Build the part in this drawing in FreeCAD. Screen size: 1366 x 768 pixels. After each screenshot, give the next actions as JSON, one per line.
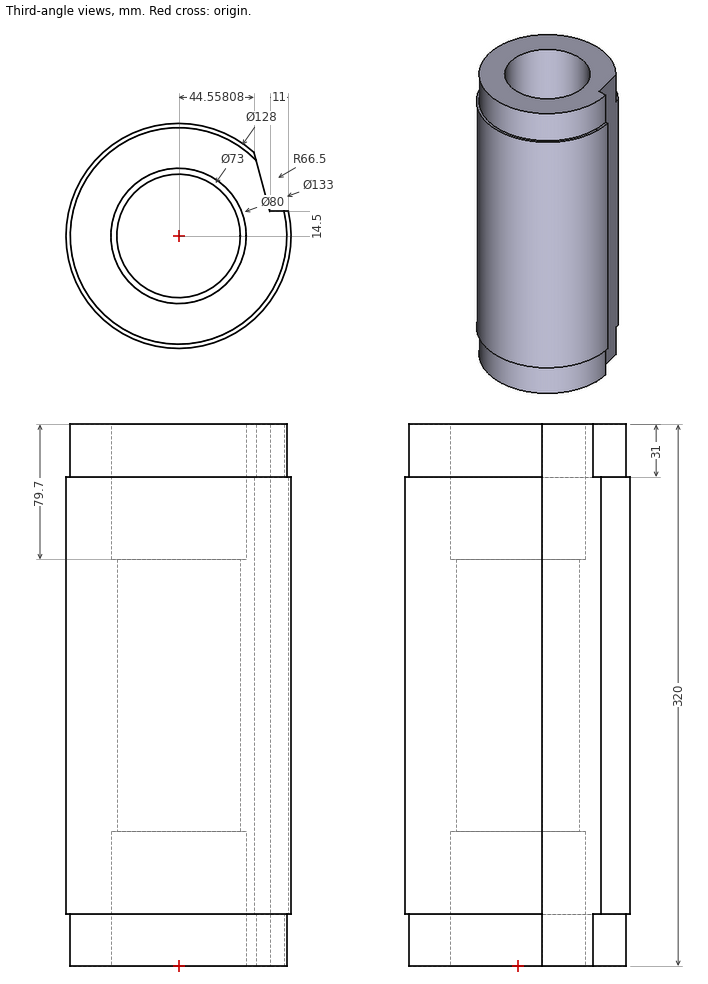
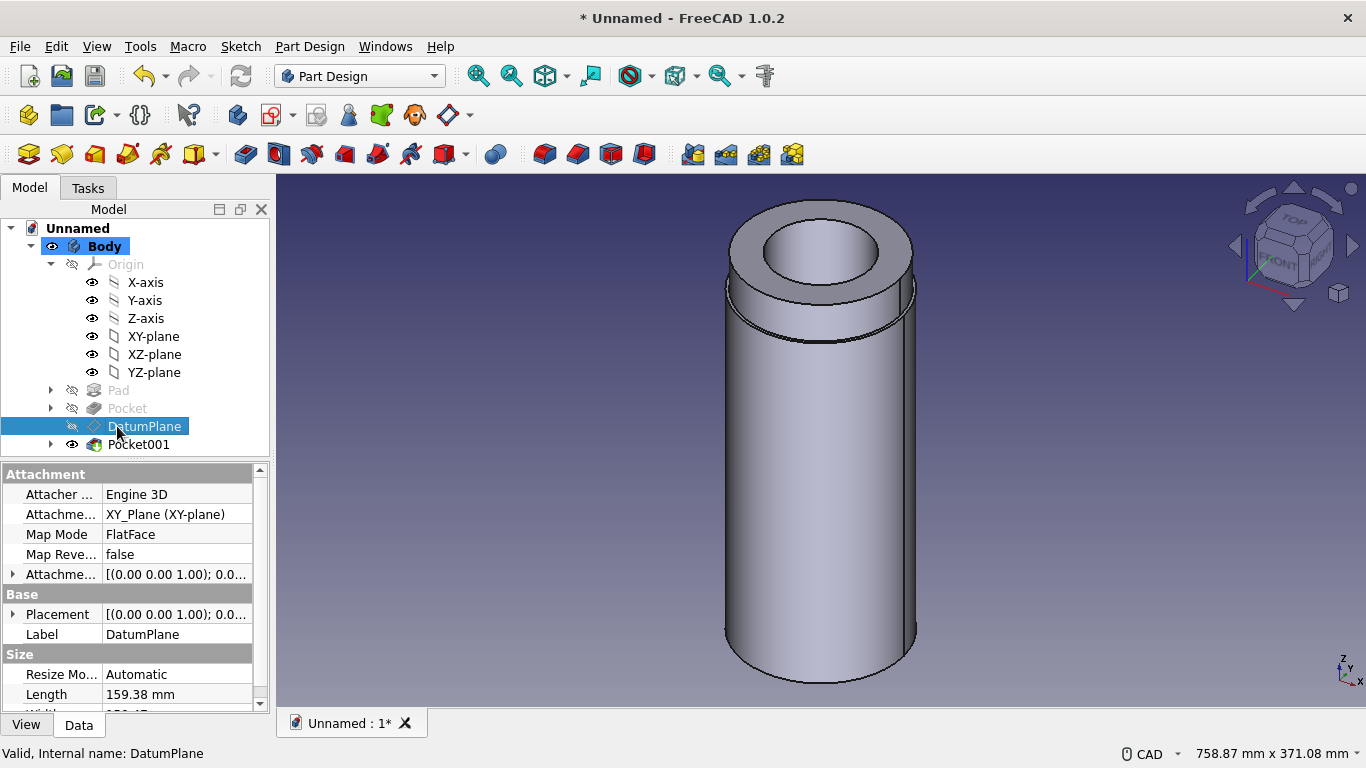
{"action": "left_click", "coordinate": [137, 336]}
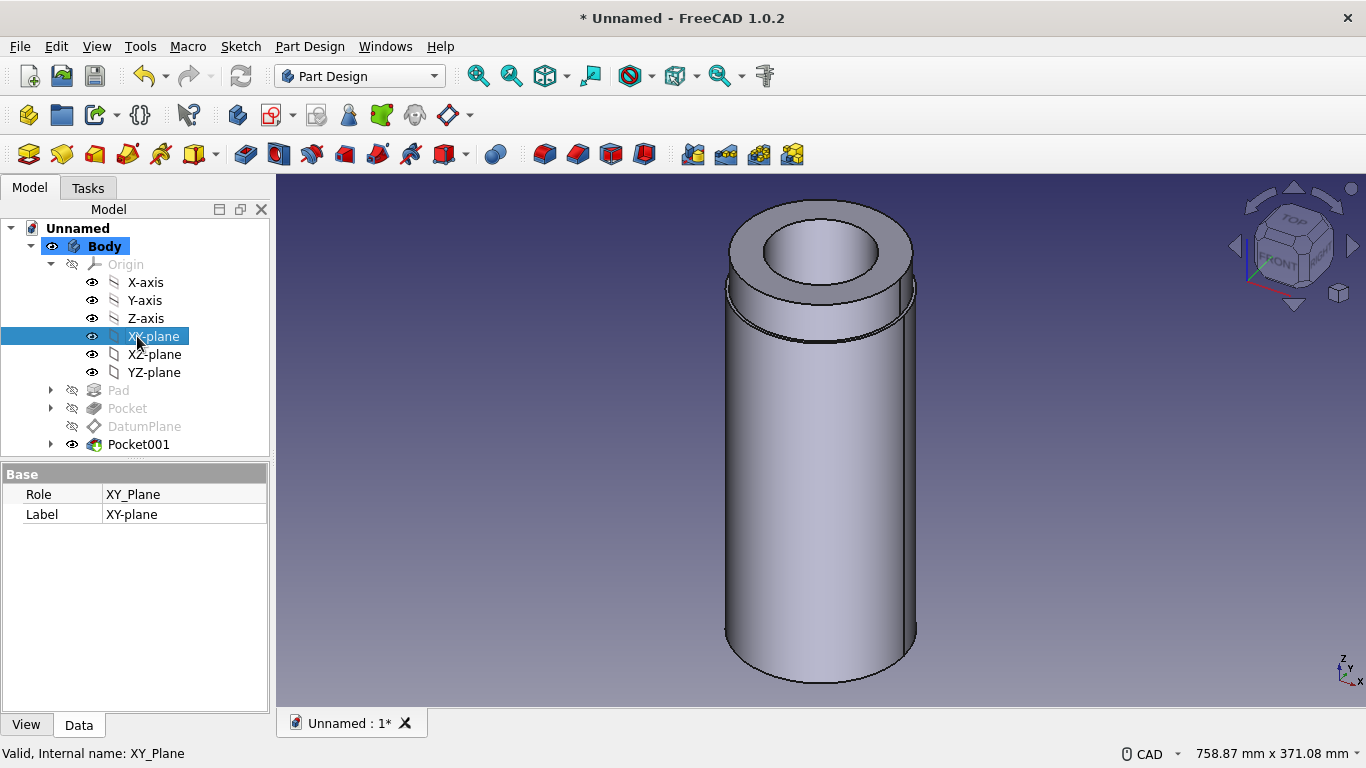
{"action": "left_click", "coordinate": [448, 116]}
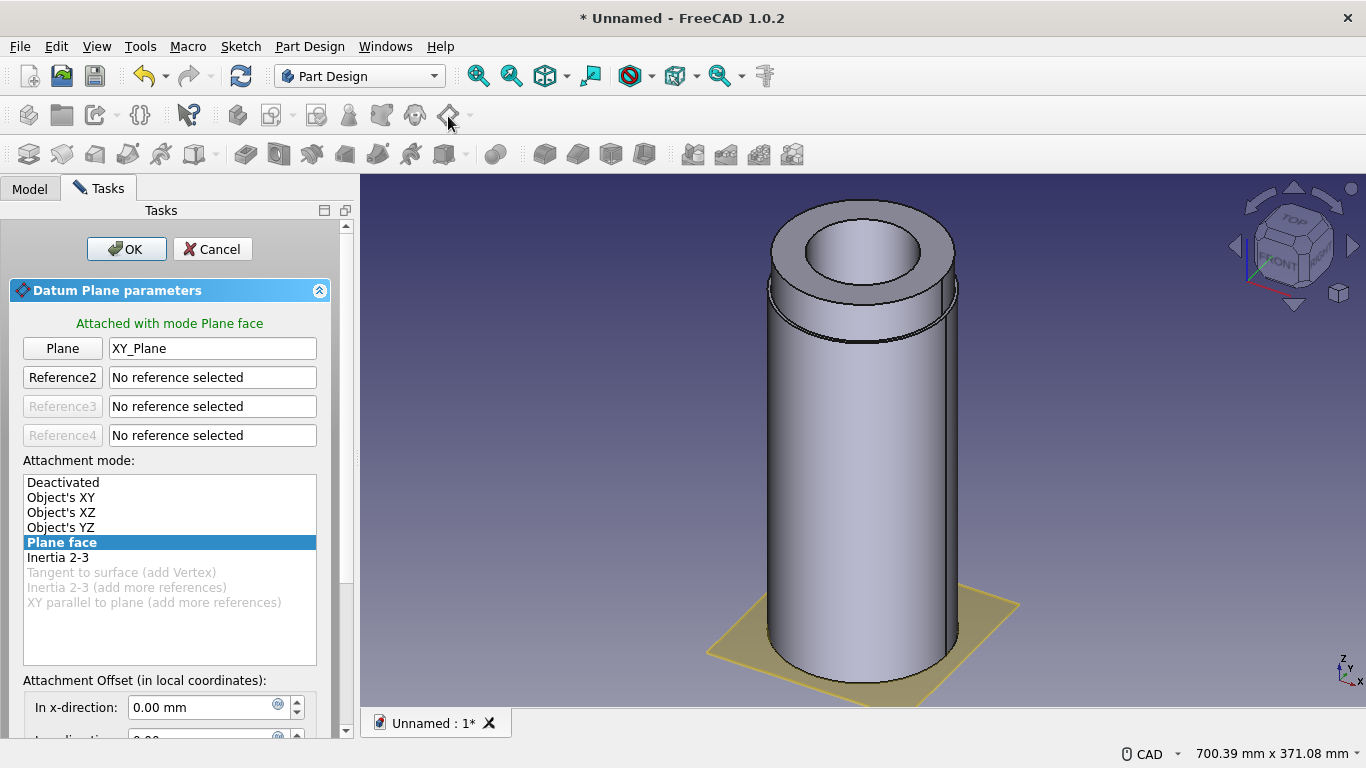
{"action": "scroll", "coordinate": [346, 479], "scroll_direction": "down", "scroll_amount": 2}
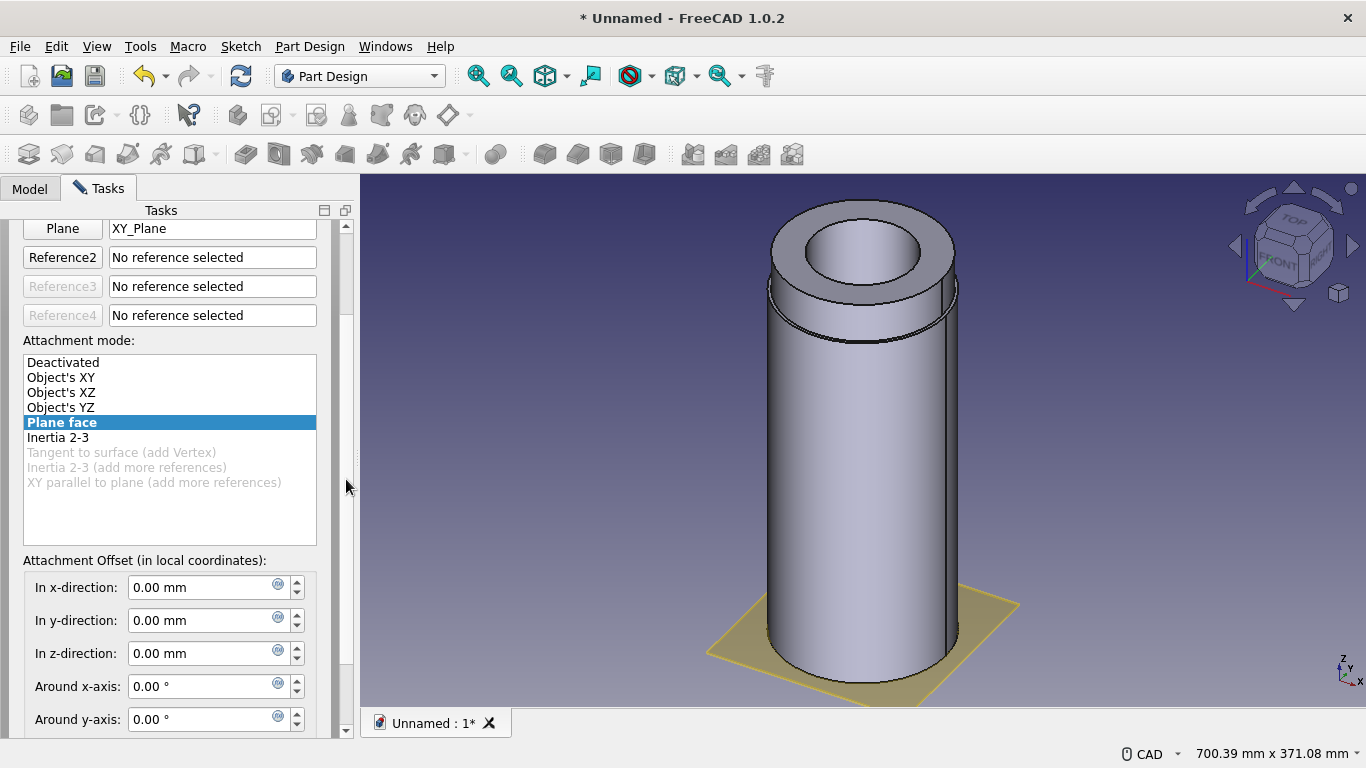
{"action": "triple_click", "coordinate": [210, 654]}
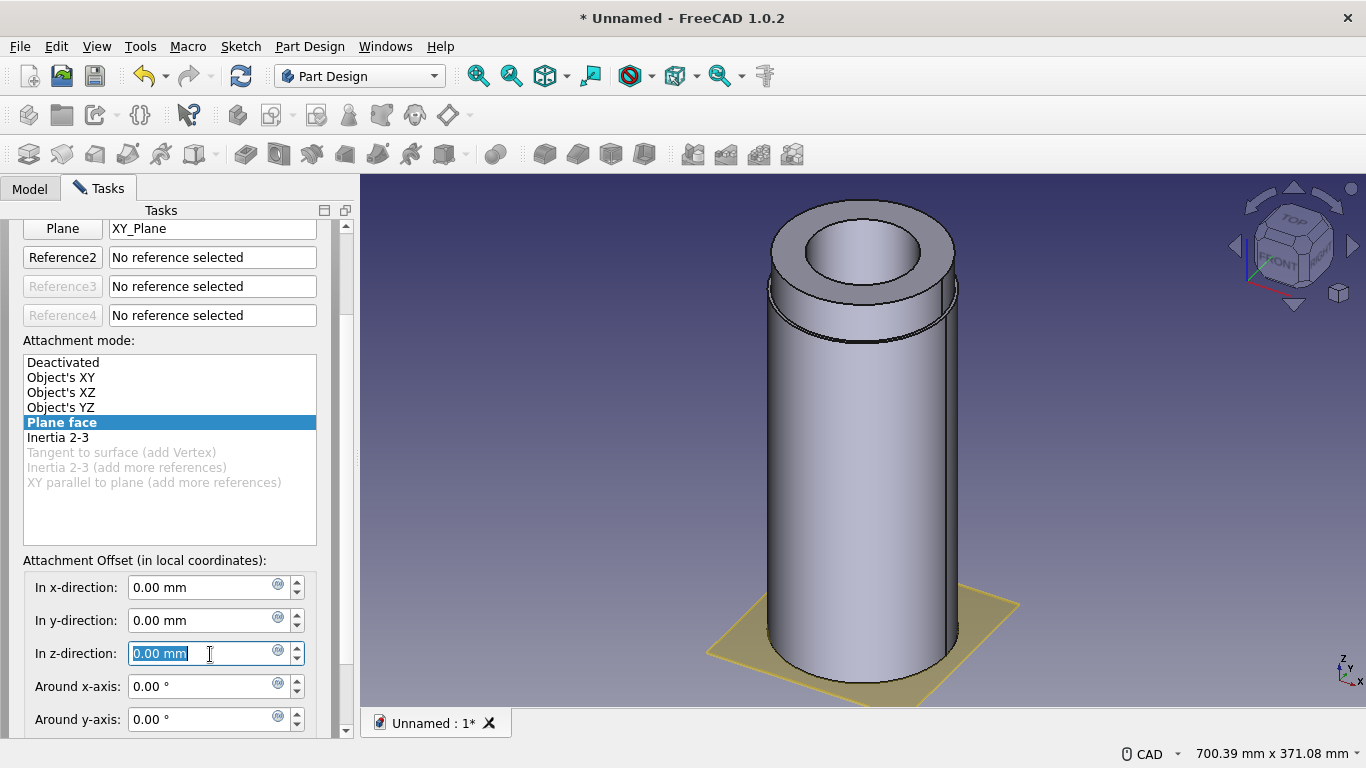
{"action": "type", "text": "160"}
{"action": "key", "text": "Tab"}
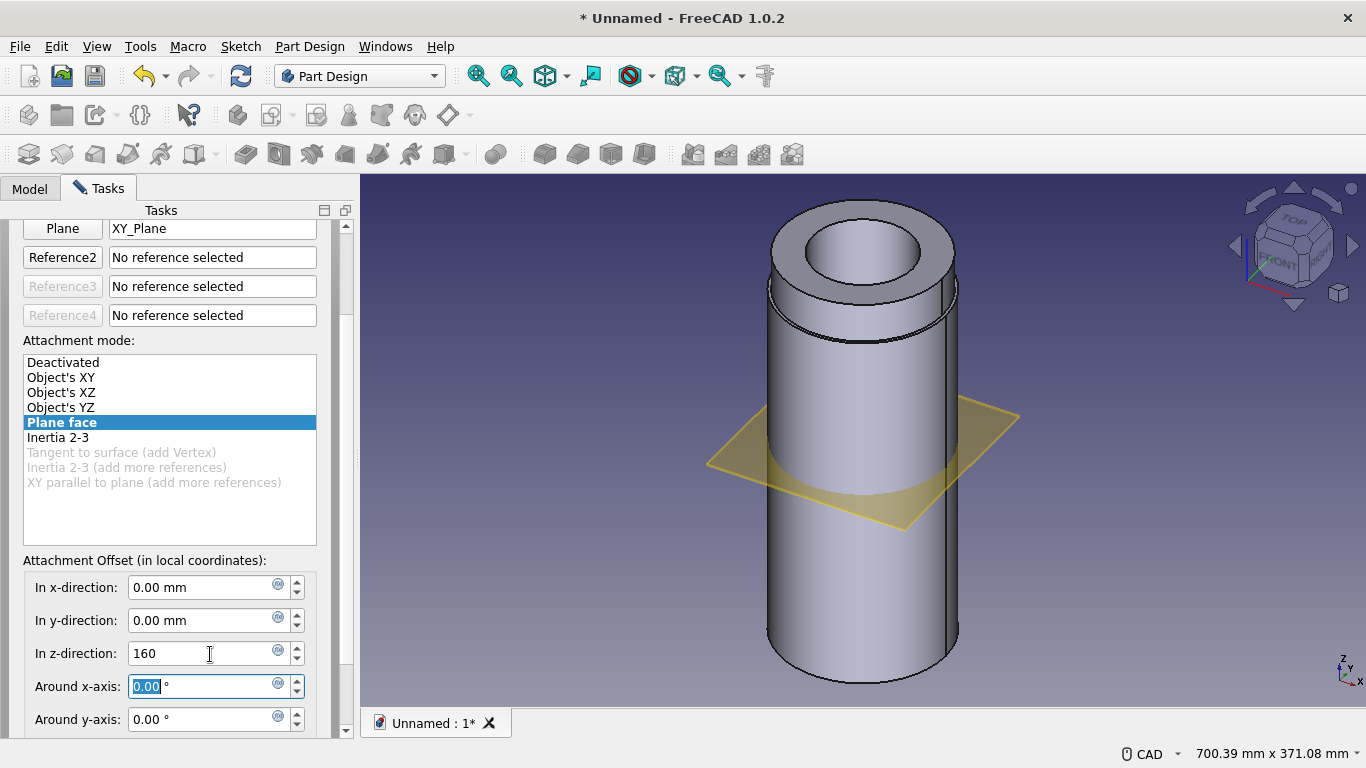
{"action": "scroll", "coordinate": [346, 479], "scroll_direction": "up", "scroll_amount": 3}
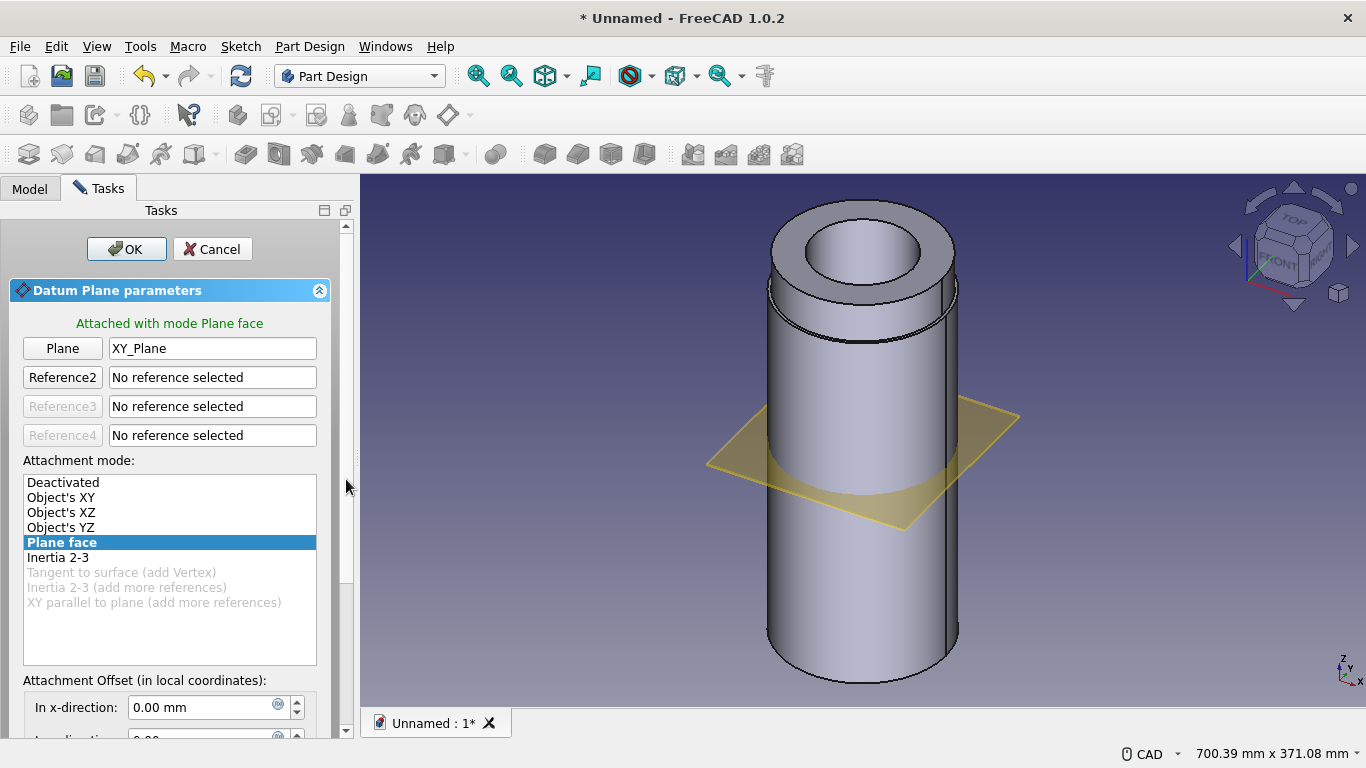
{"action": "left_click", "coordinate": [127, 249]}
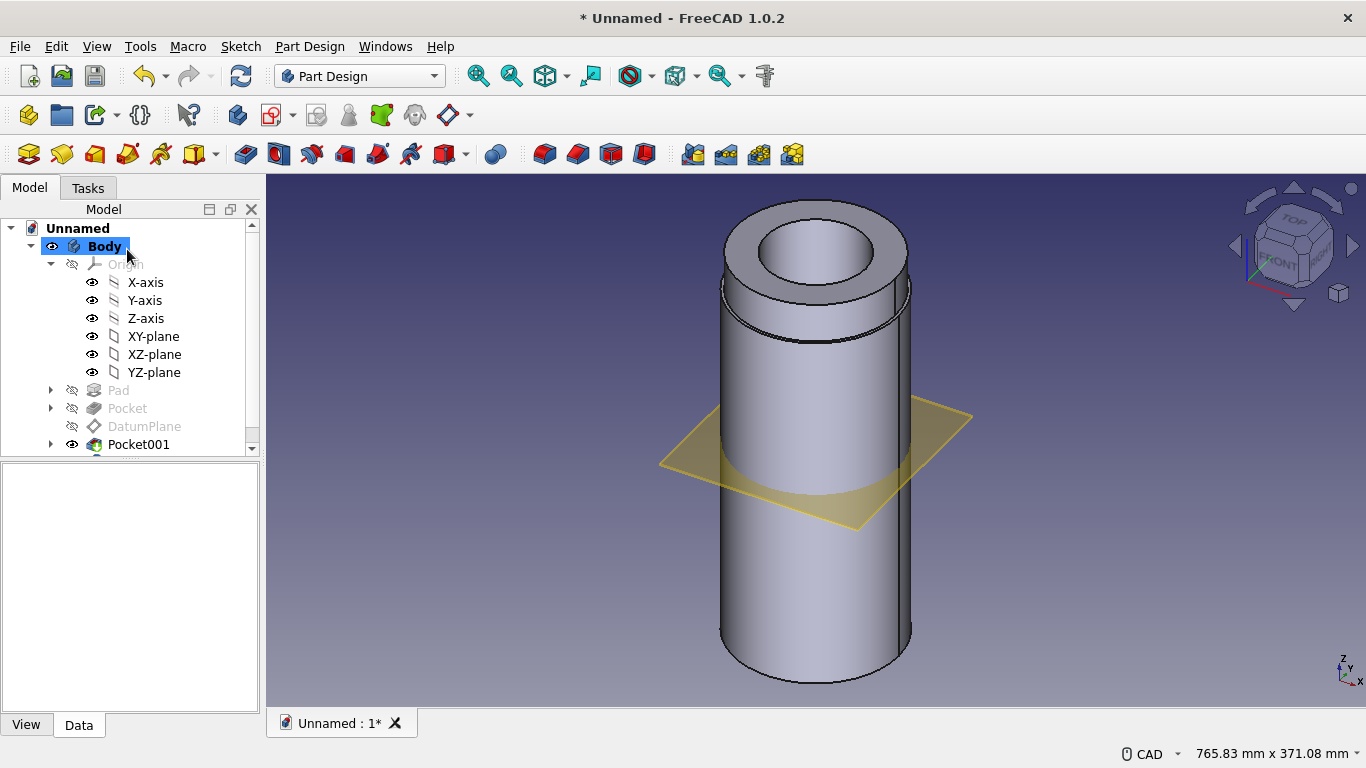
{"action": "left_click", "coordinate": [117, 408]}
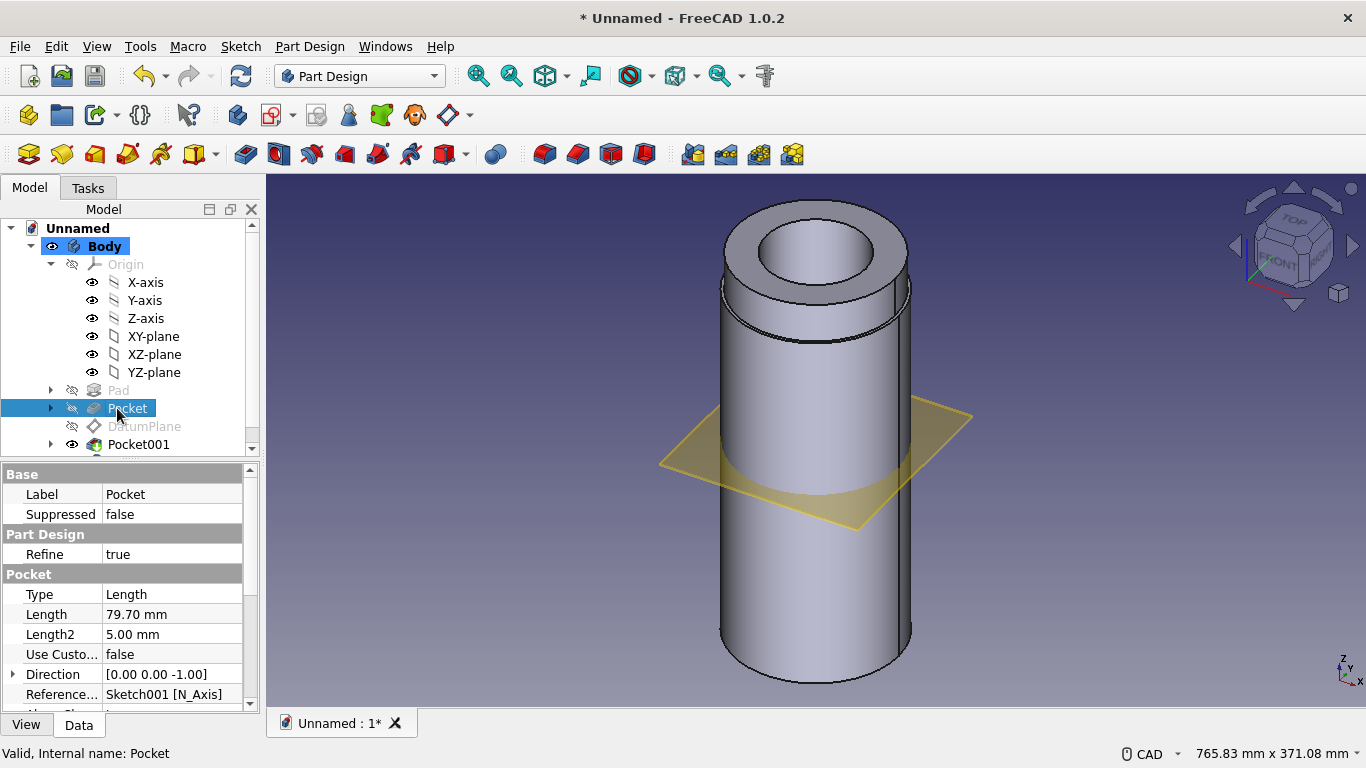
{"action": "left_click", "coordinate": [117, 444], "text": "ctrl"}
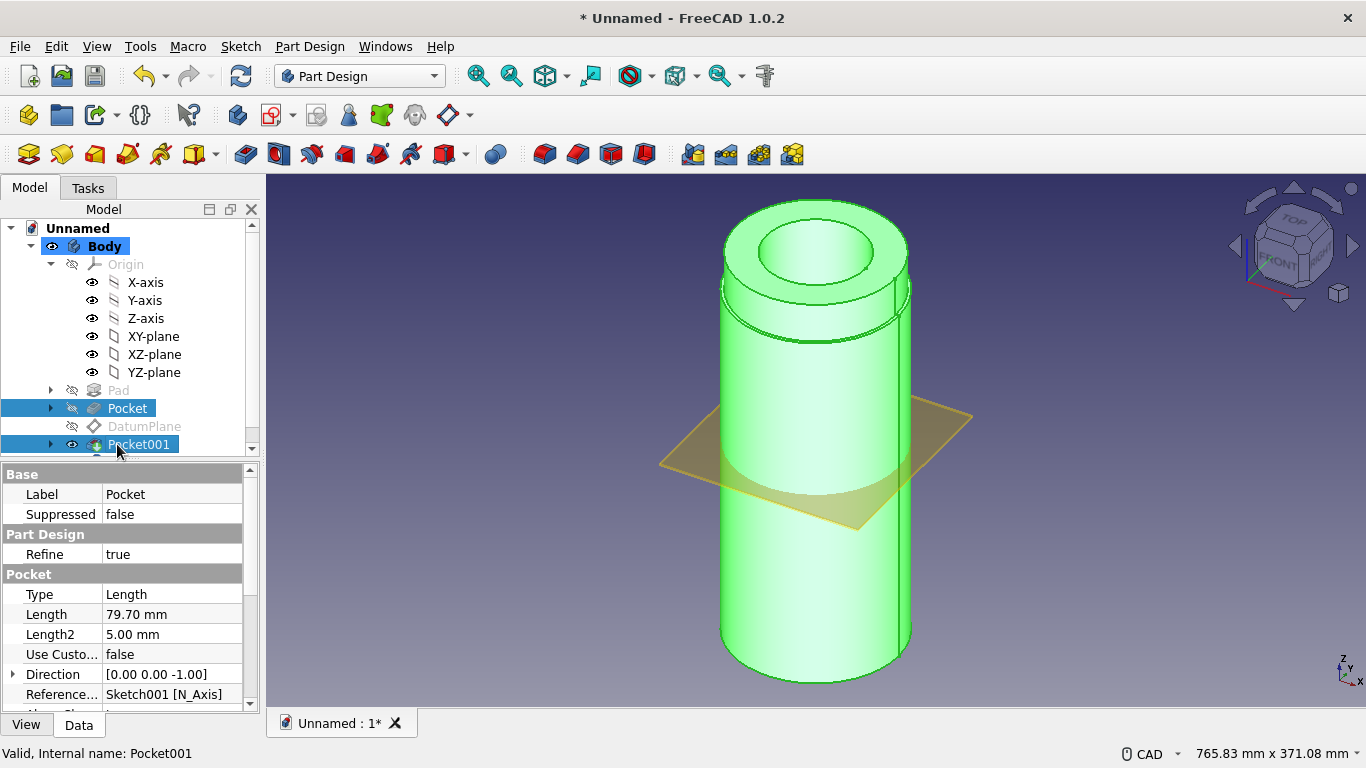
{"action": "left_click", "coordinate": [693, 154]}